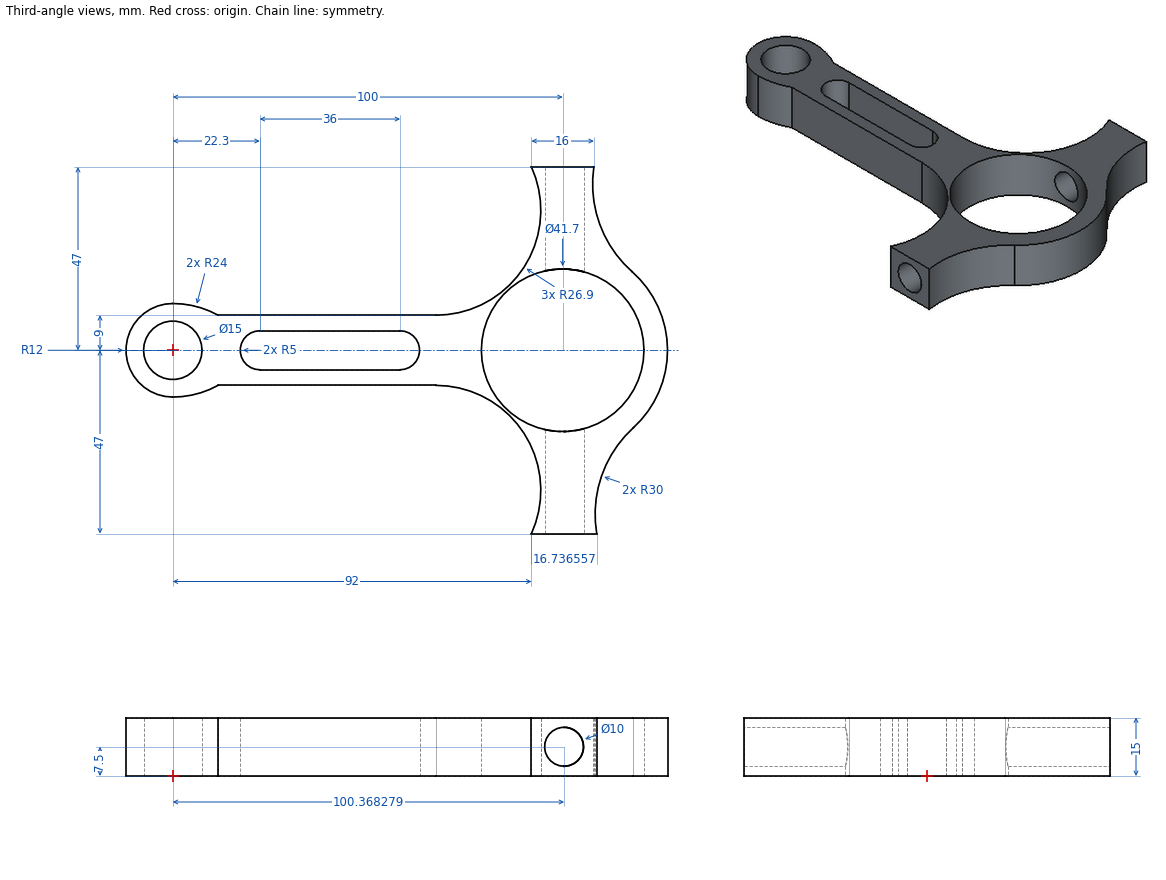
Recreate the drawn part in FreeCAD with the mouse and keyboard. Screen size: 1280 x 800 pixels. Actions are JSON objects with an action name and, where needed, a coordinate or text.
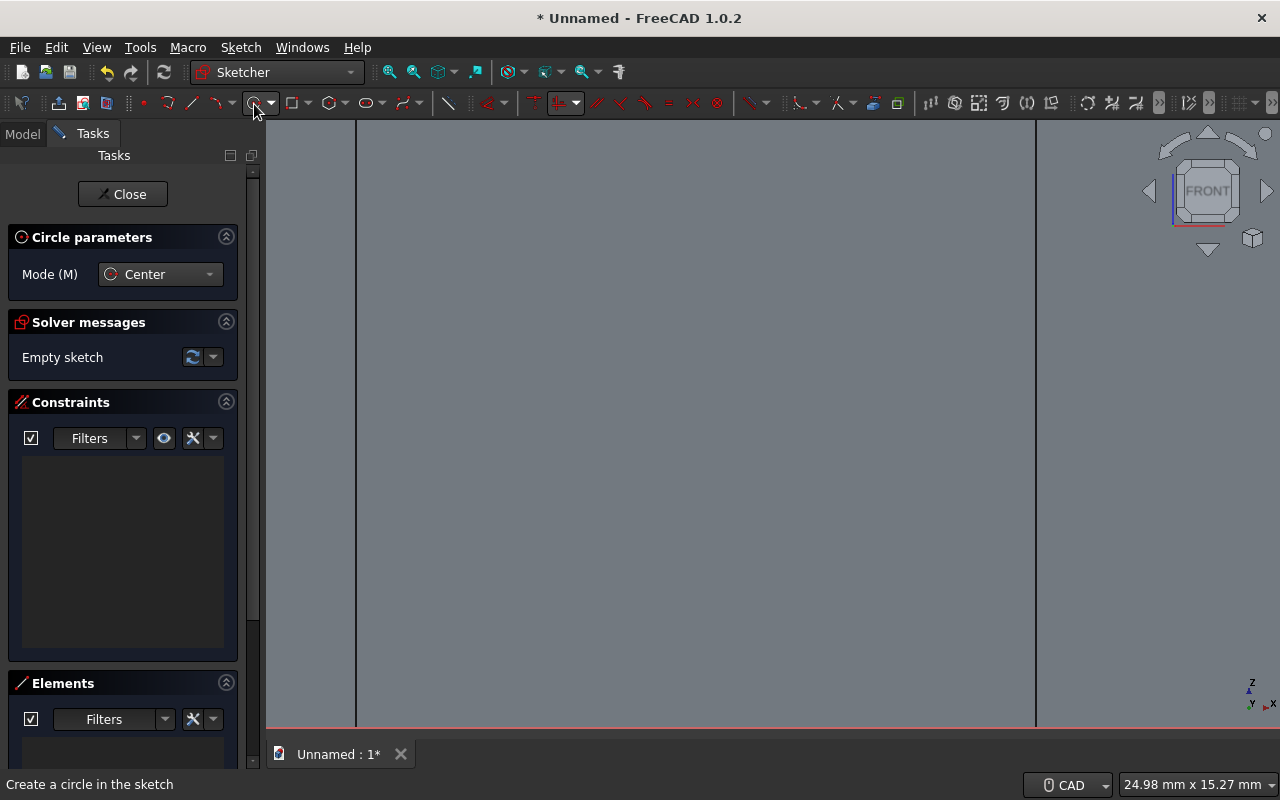
{"action": "left_click", "coordinate": [696, 424]}
{"action": "left_click", "coordinate": [839, 280]}
{"action": "key", "text": "Escape"}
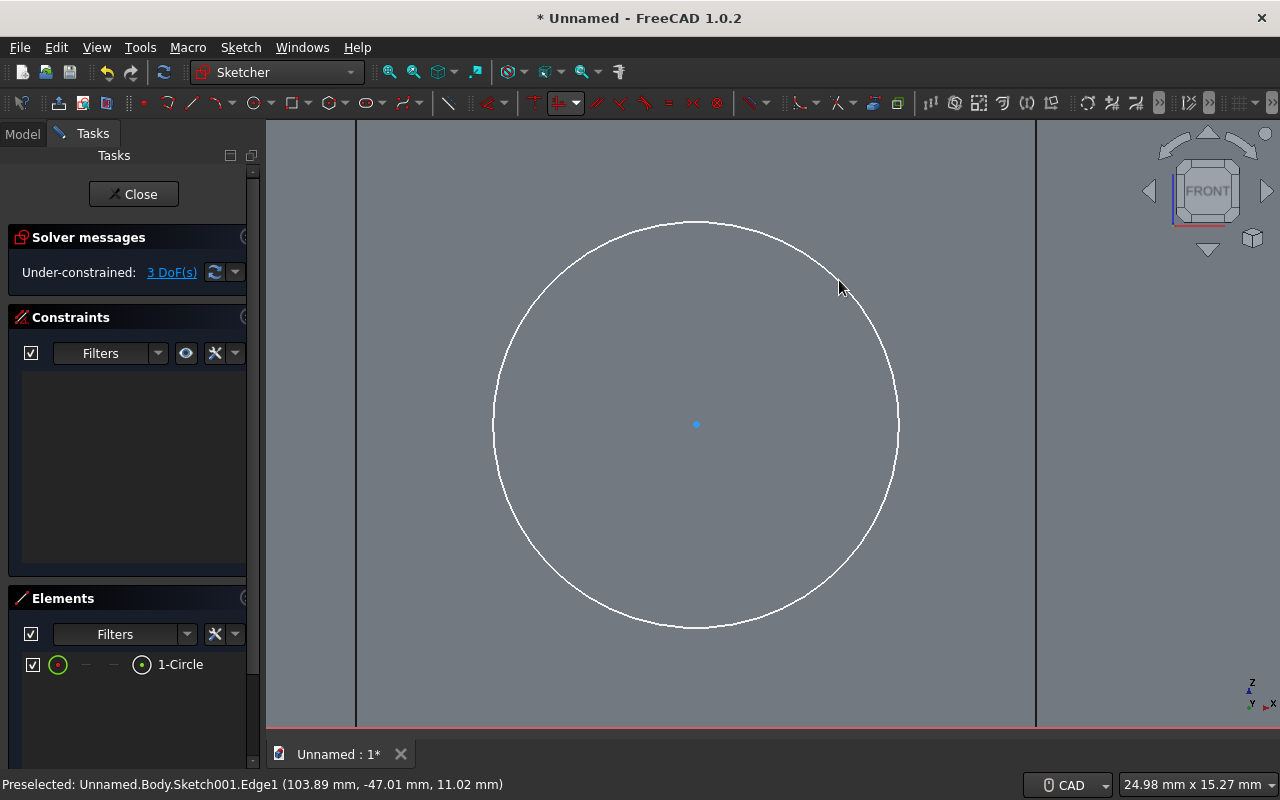
{"action": "left_click", "coordinate": [488, 104]}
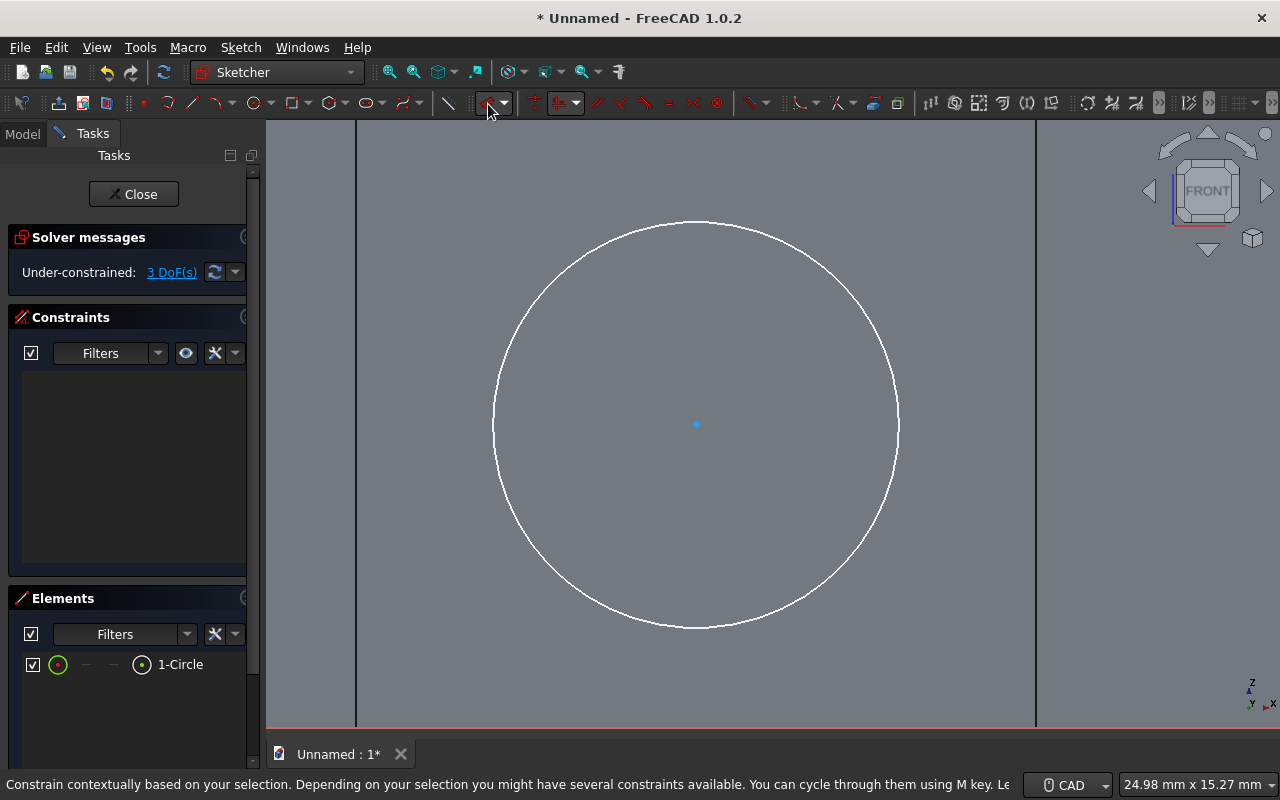
{"action": "left_click", "coordinate": [839, 281]}
{"action": "left_click", "coordinate": [862, 258]}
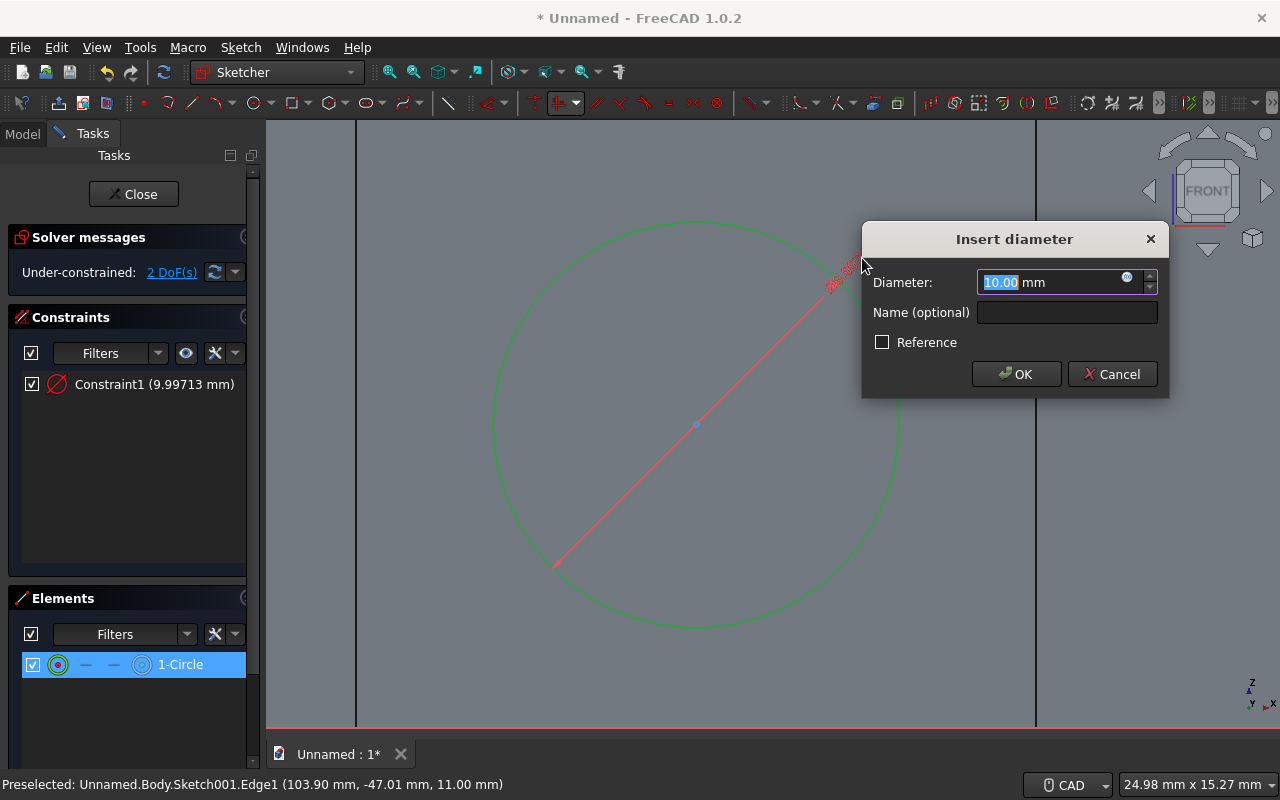
{"action": "type", "text": "10"}
{"action": "key", "text": "Return"}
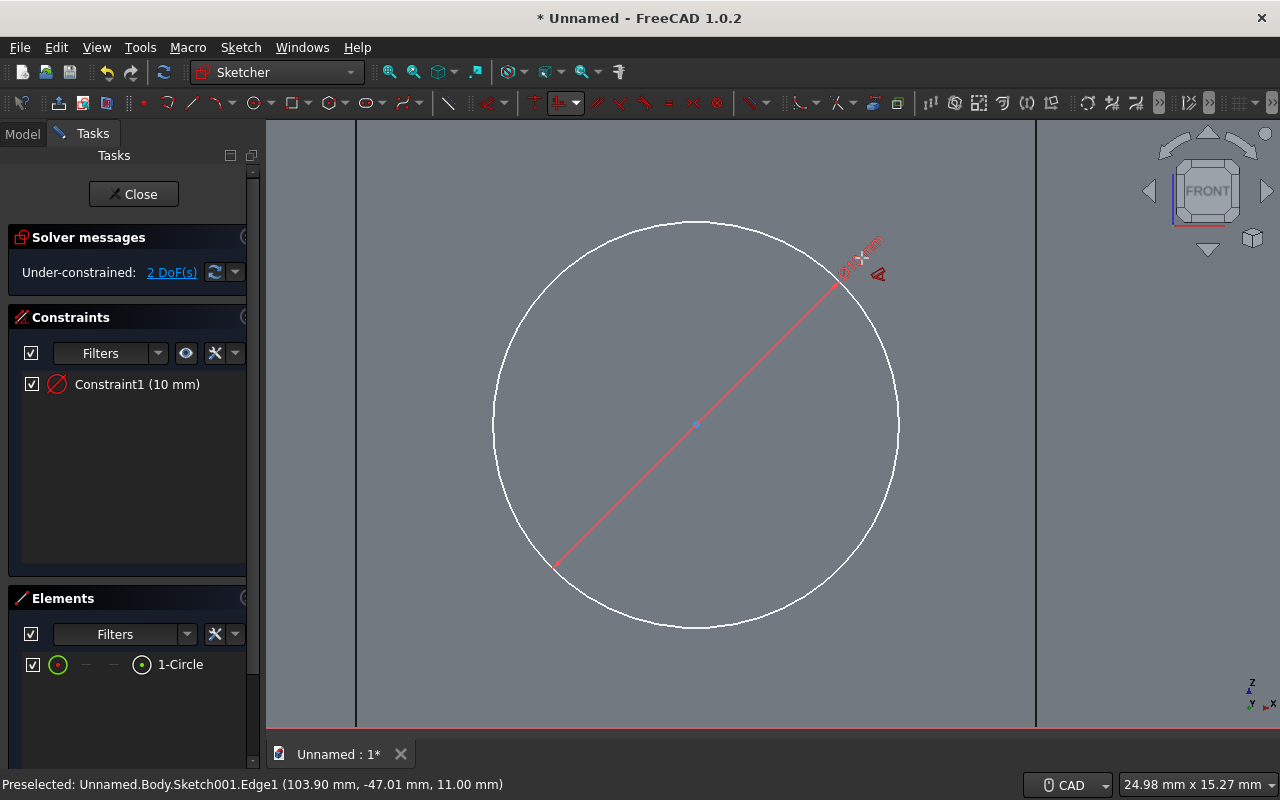
{"action": "left_click", "coordinate": [696, 425]}
{"action": "left_click", "coordinate": [730, 568]}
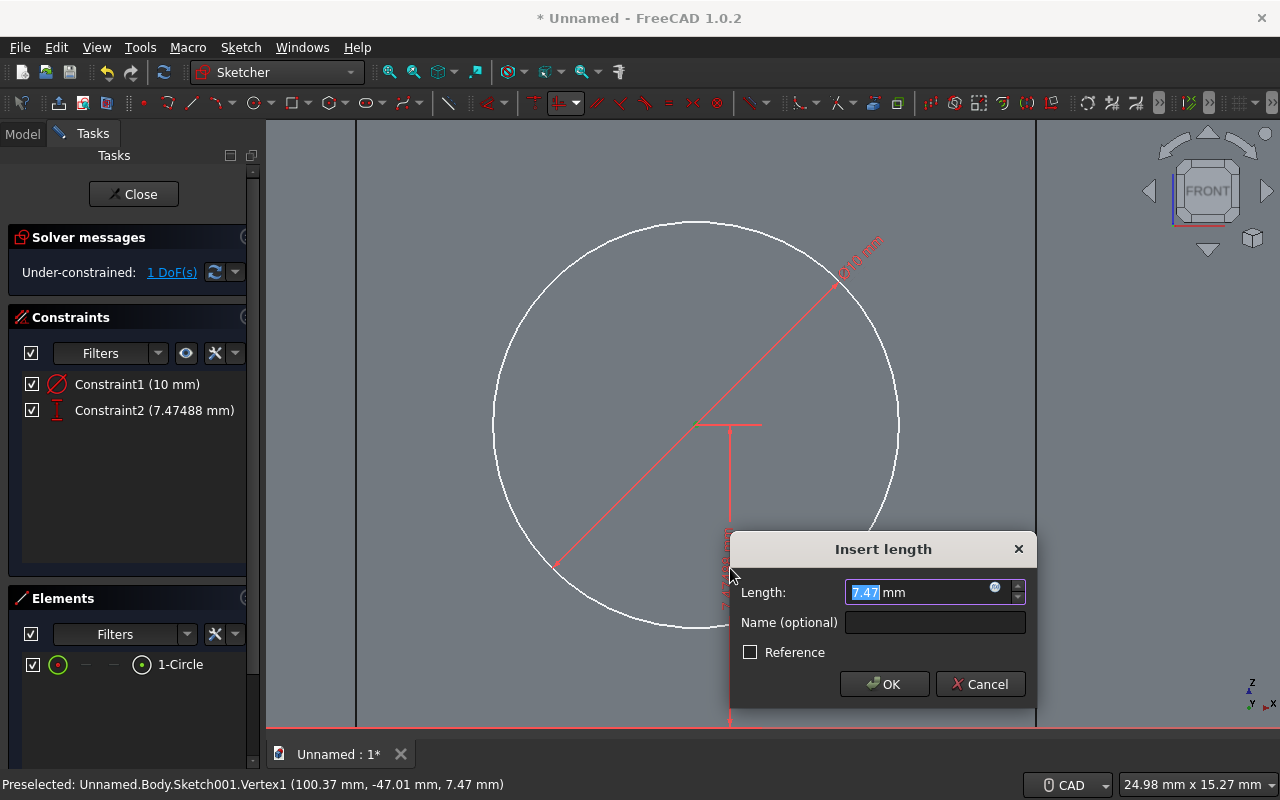
{"action": "type", "text": "7.5"}
{"action": "key", "text": "Return"}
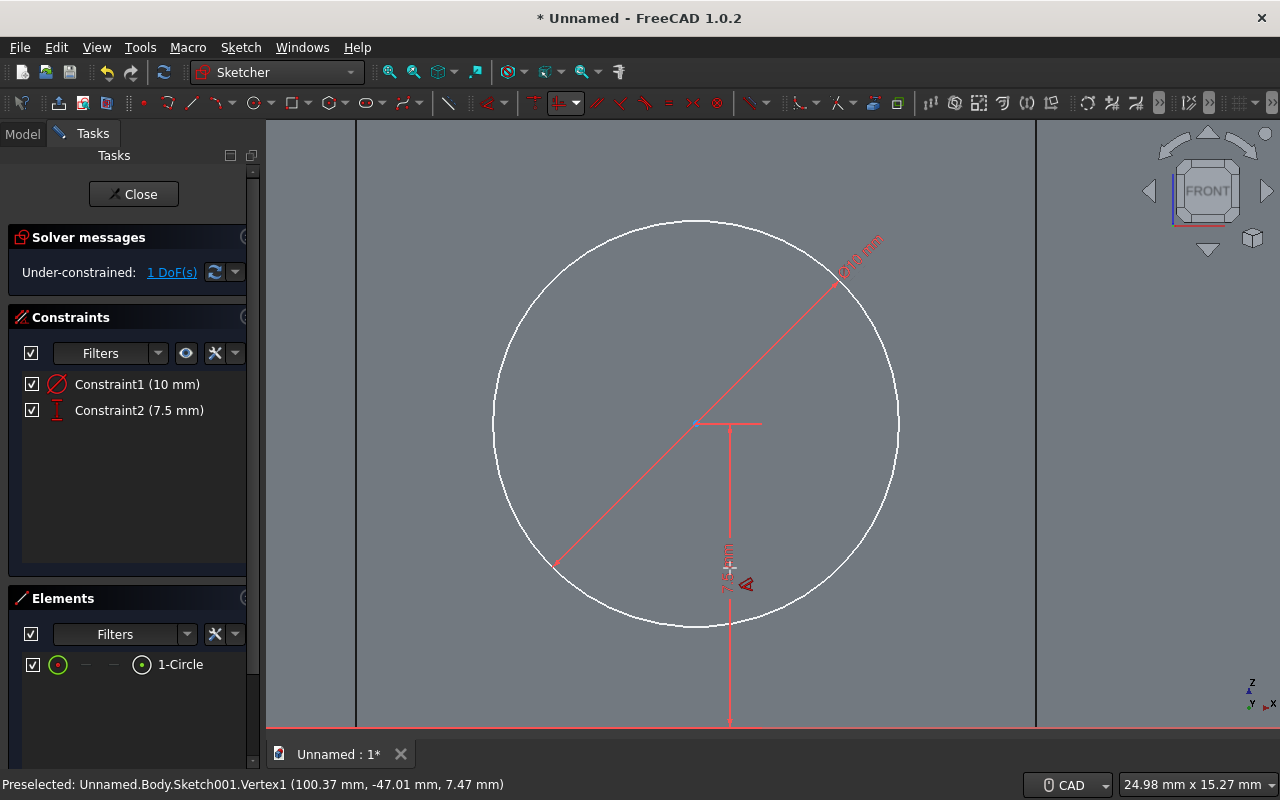
{"action": "left_click", "coordinate": [696, 424]}
{"action": "left_click", "coordinate": [403, 390]}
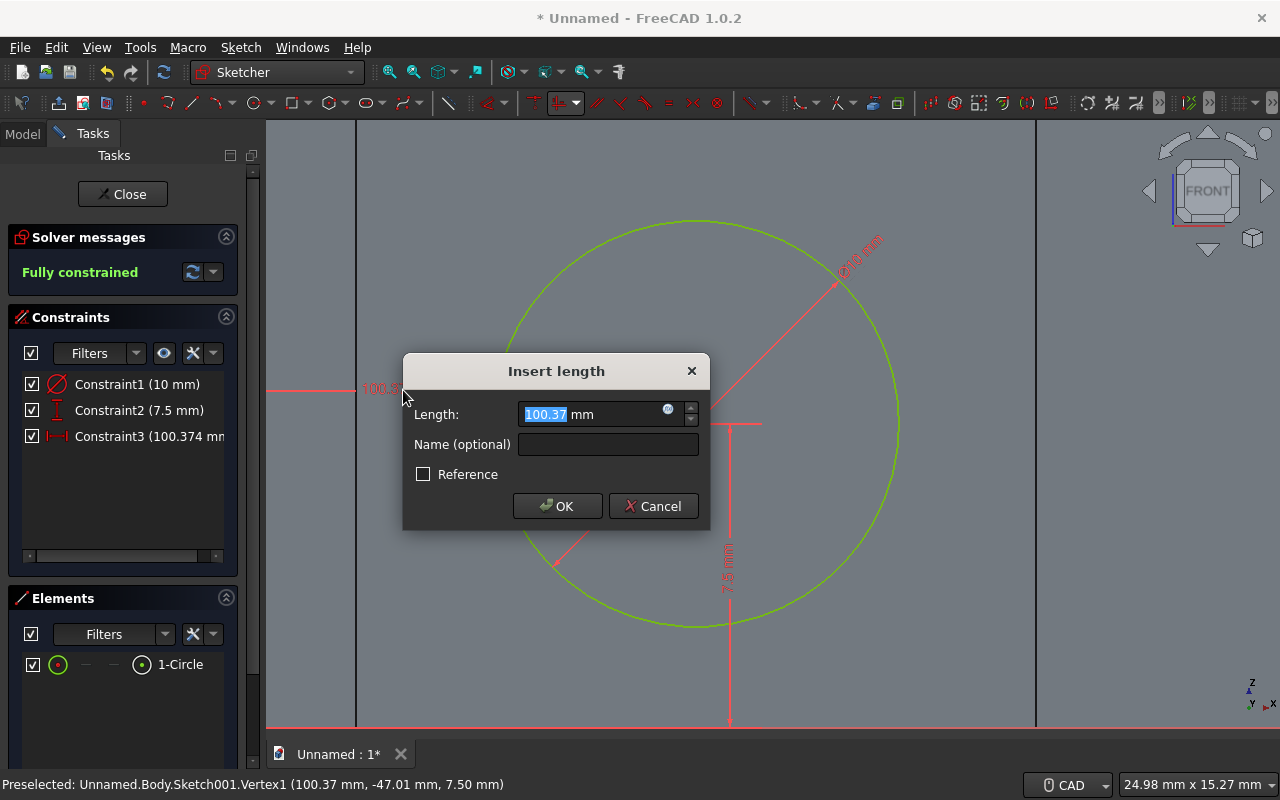
{"action": "type", "text": "100.368279"}
{"action": "key", "text": "Return"}
{"action": "key", "text": "Escape"}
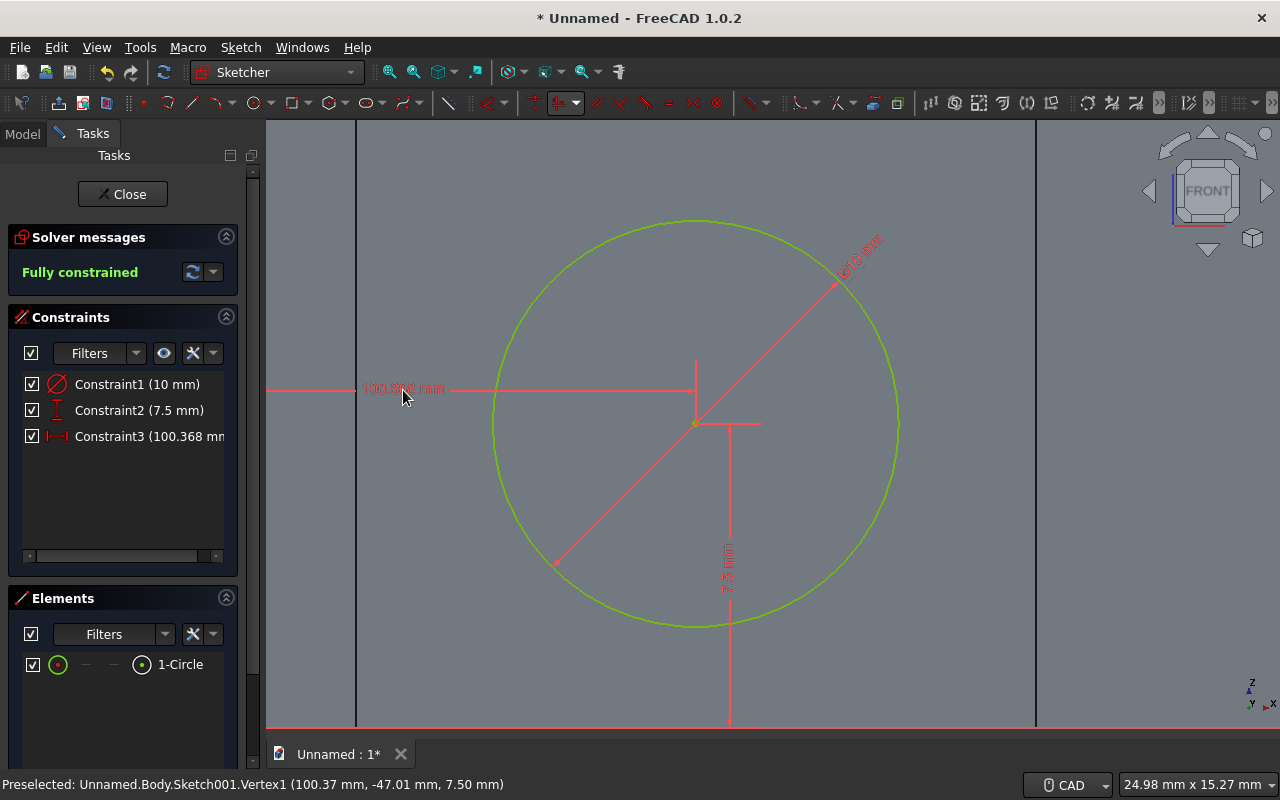
{"action": "left_click", "coordinate": [123, 194]}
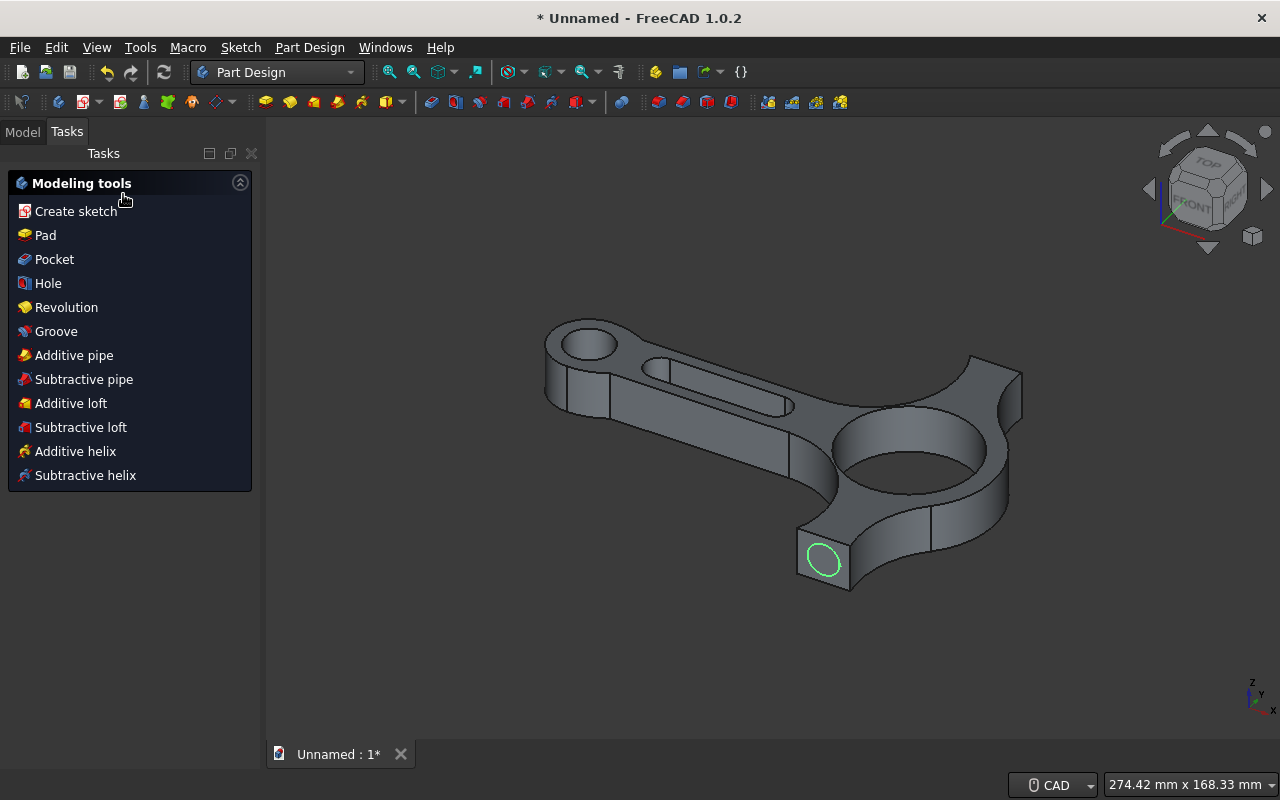
{"action": "left_click", "coordinate": [432, 102]}